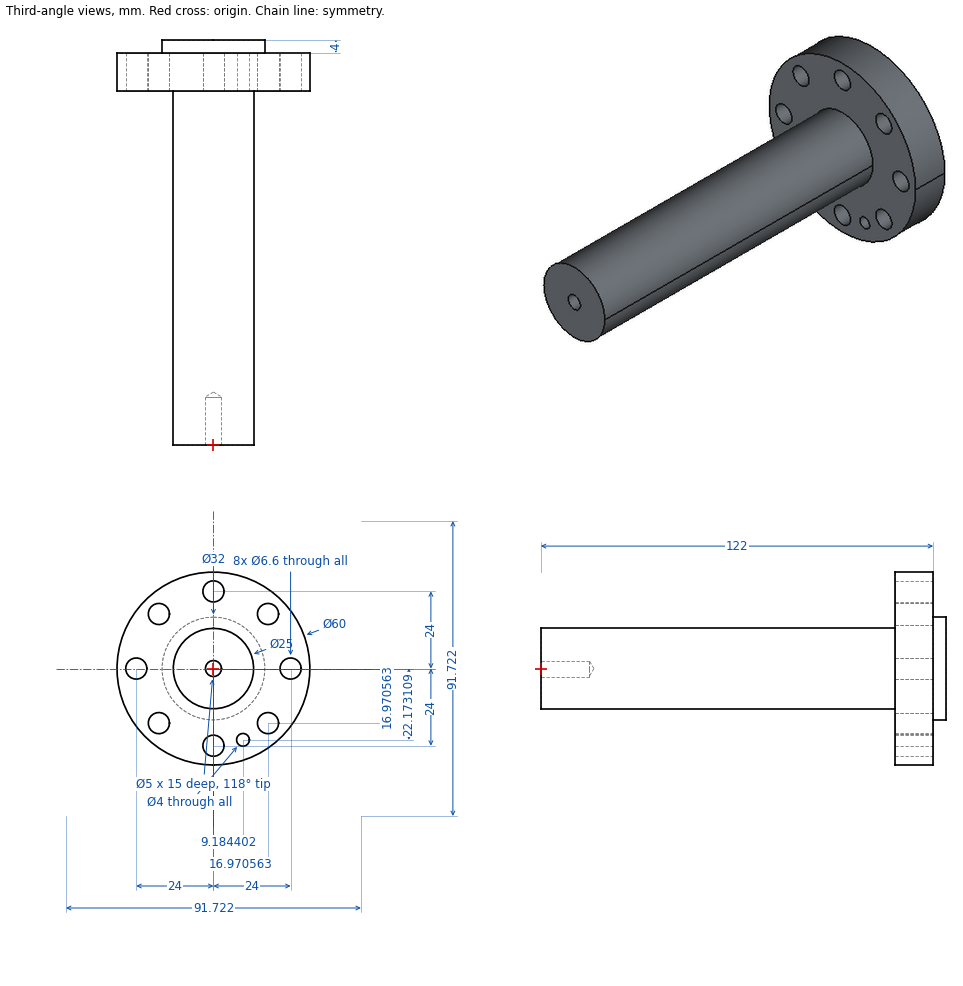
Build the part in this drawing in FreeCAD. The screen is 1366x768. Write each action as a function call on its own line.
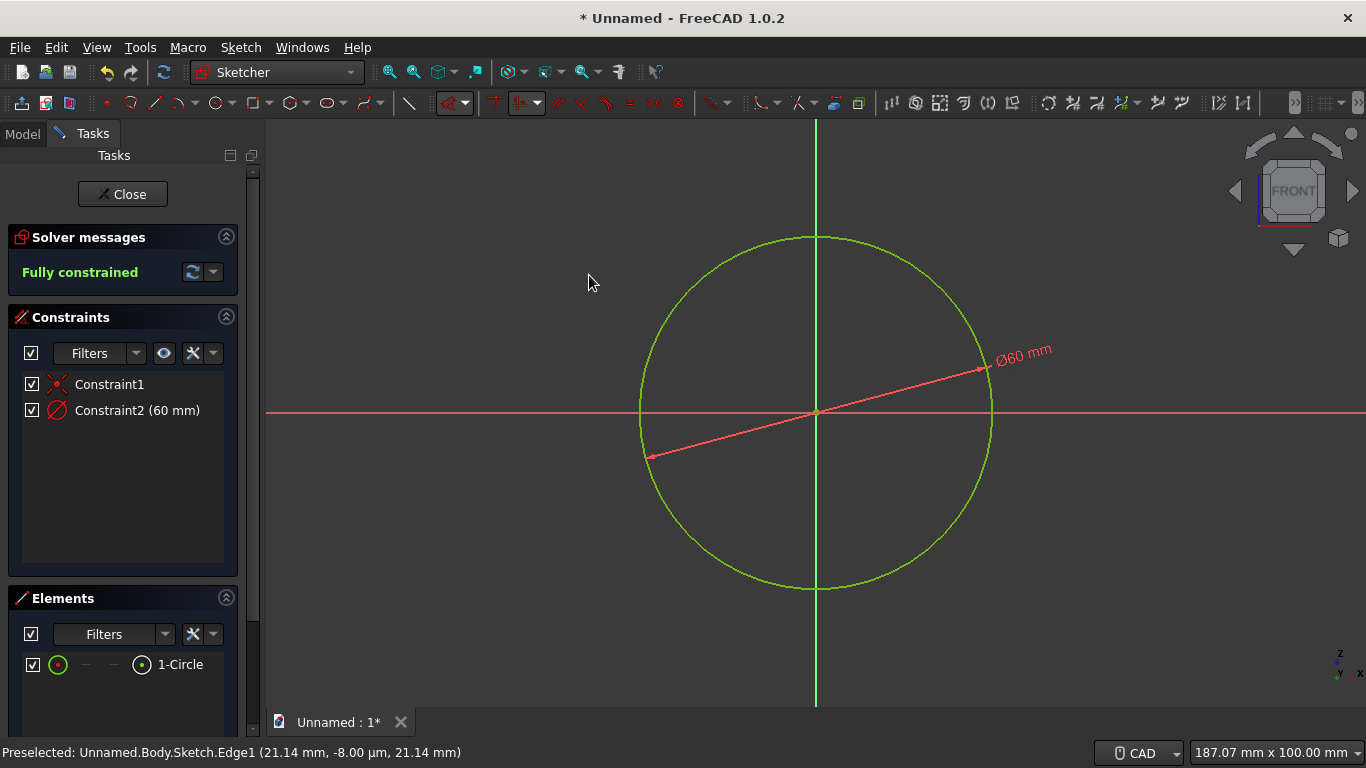
click(123, 194)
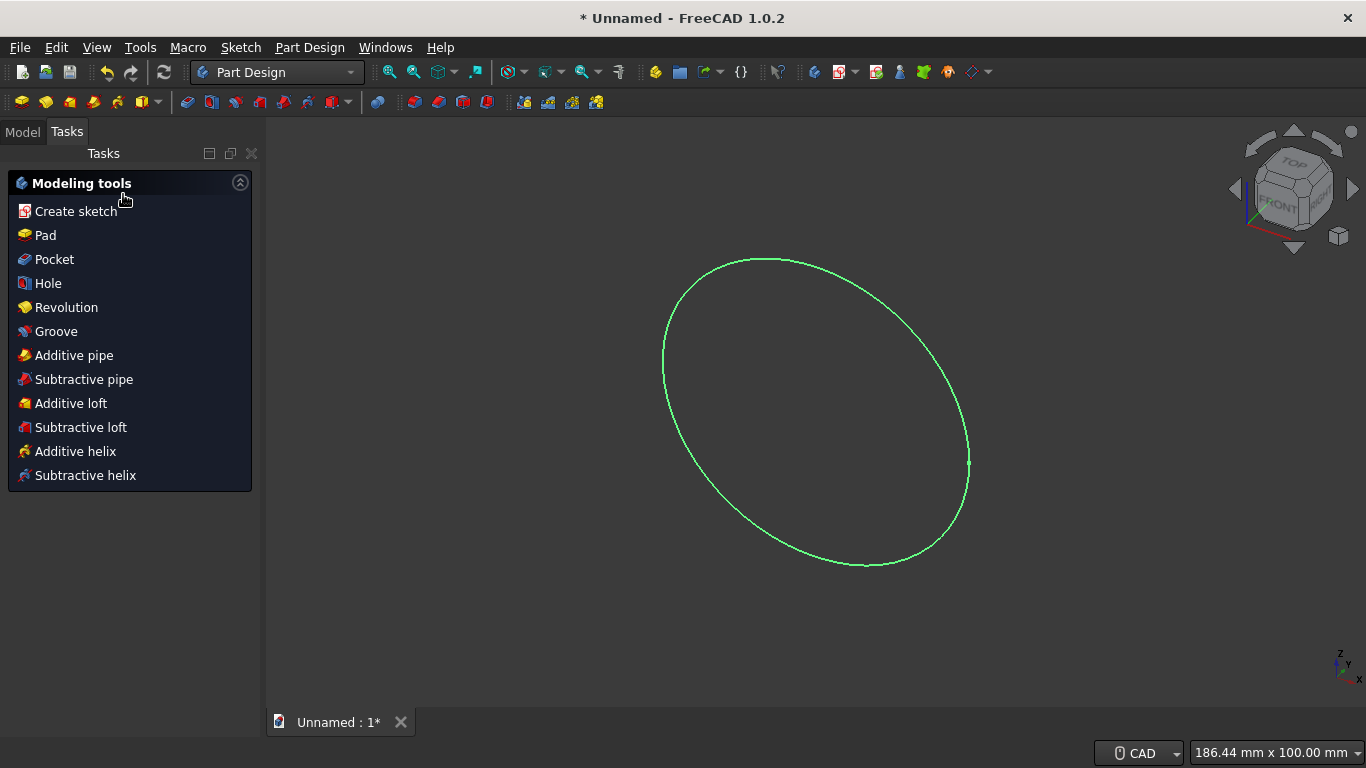
click(22, 102)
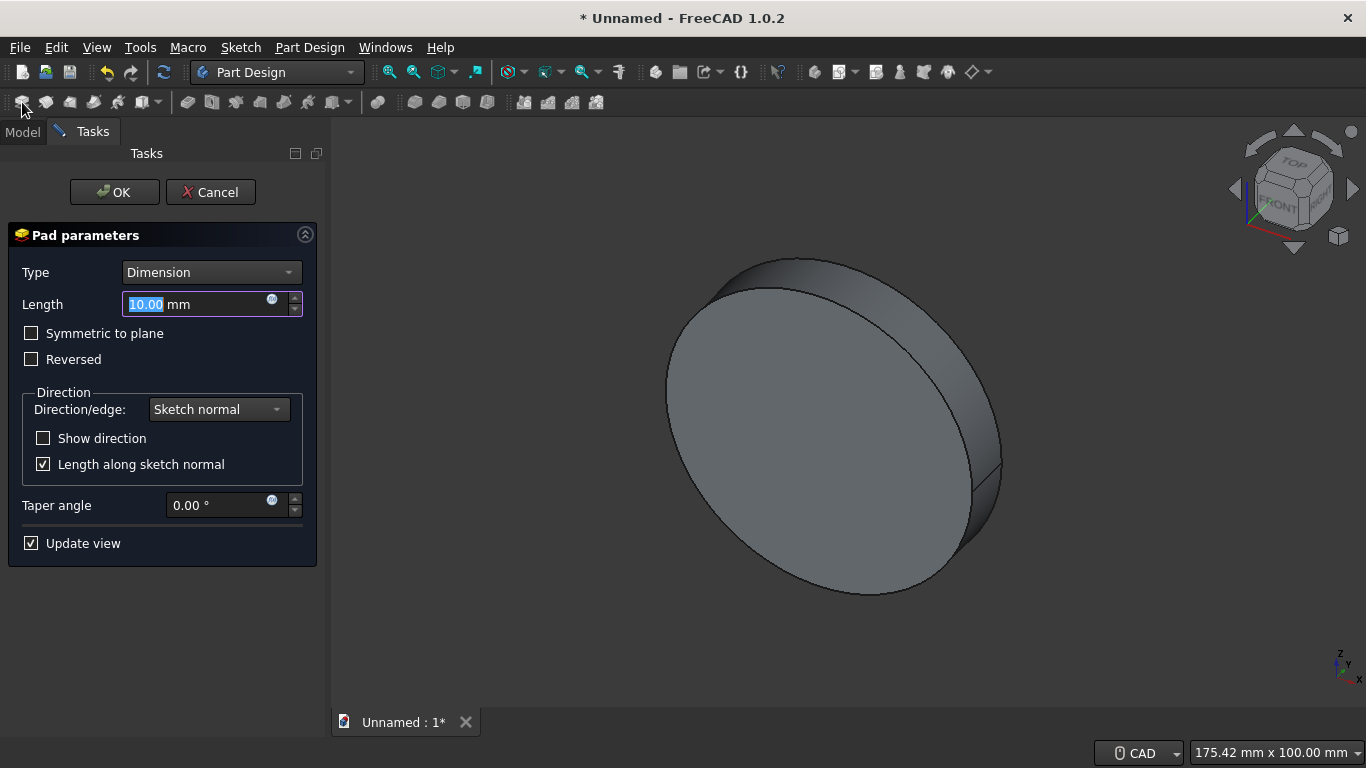
text(122)
key(Tab)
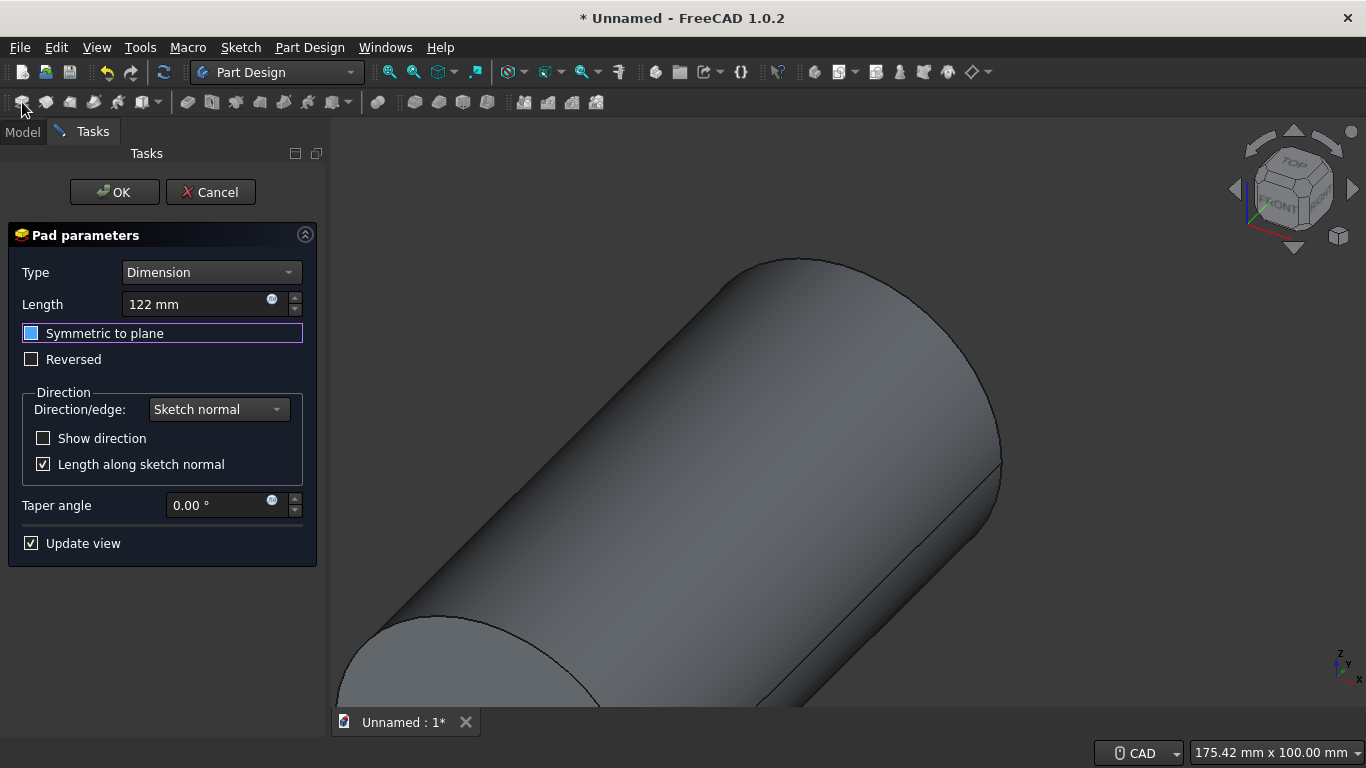
click(30, 359)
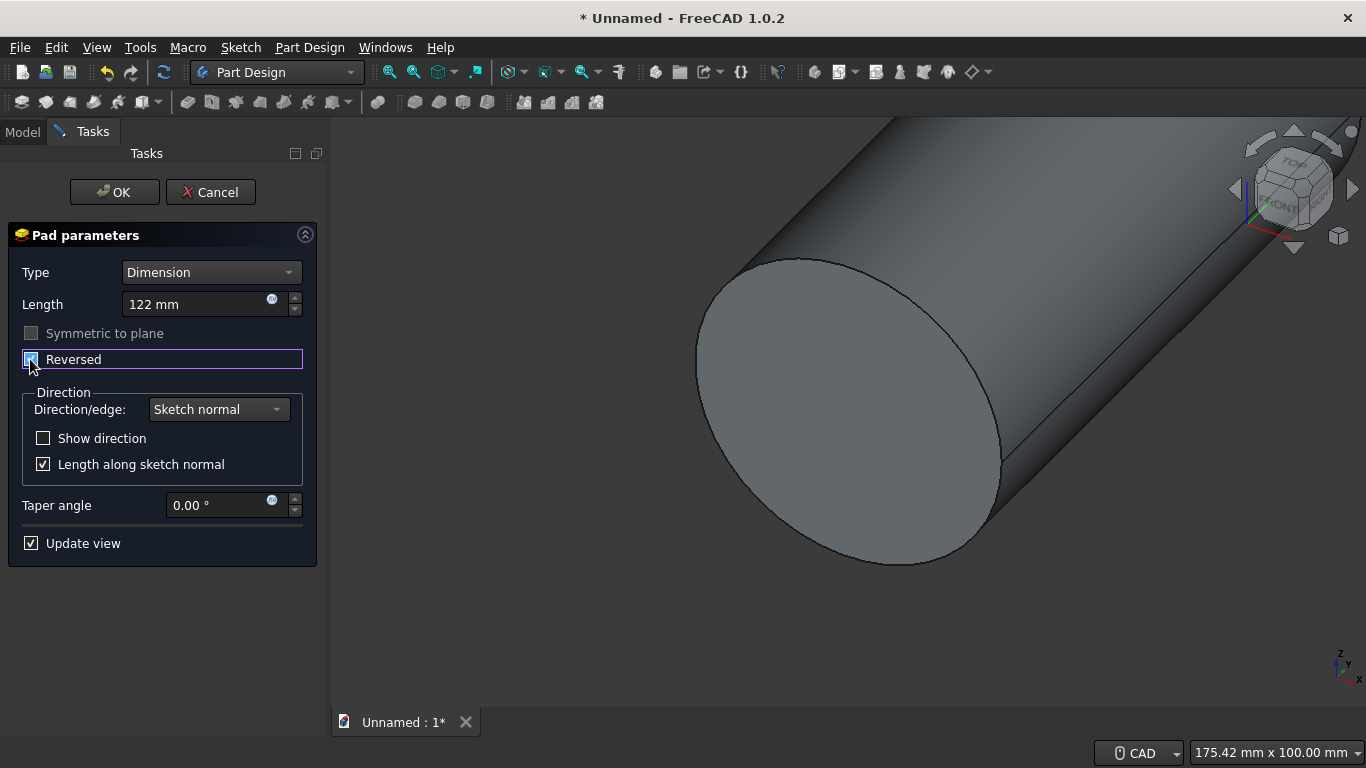
click(115, 192)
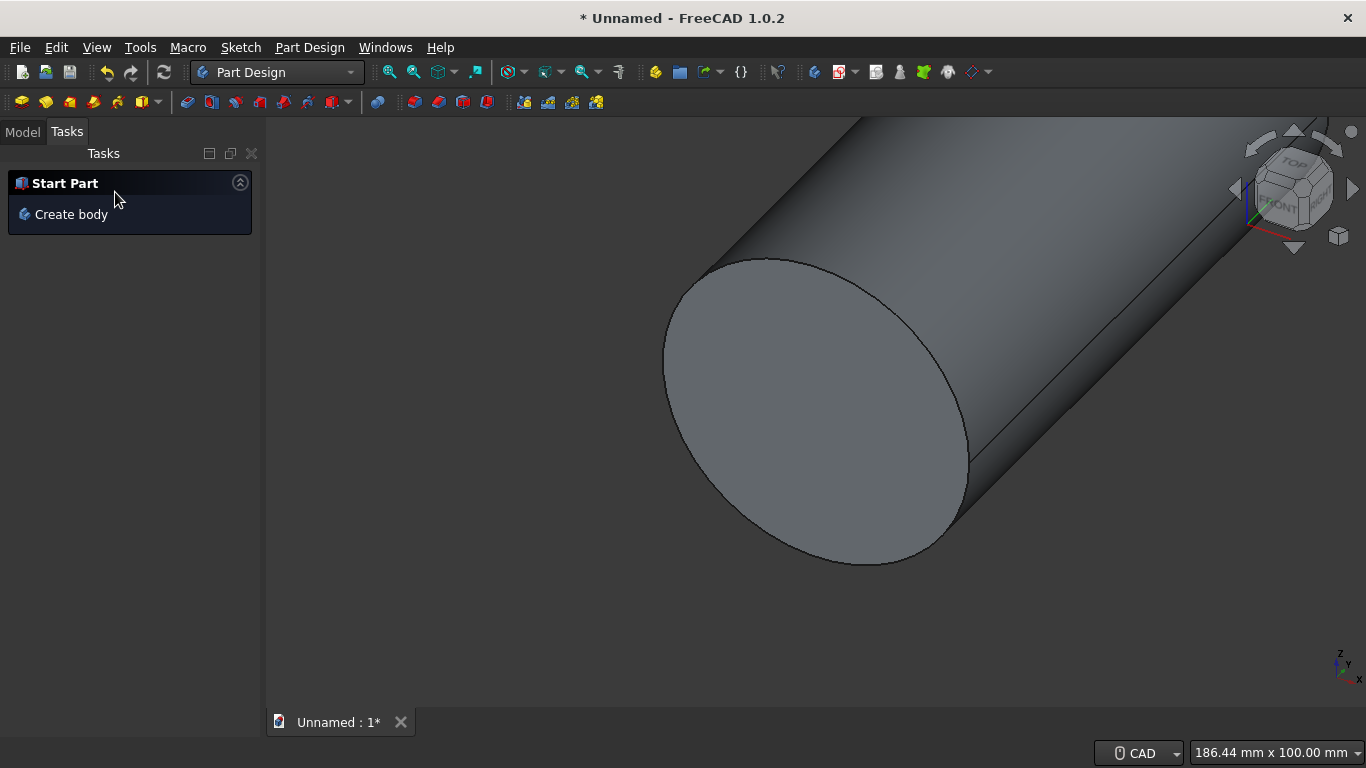
click(390, 72)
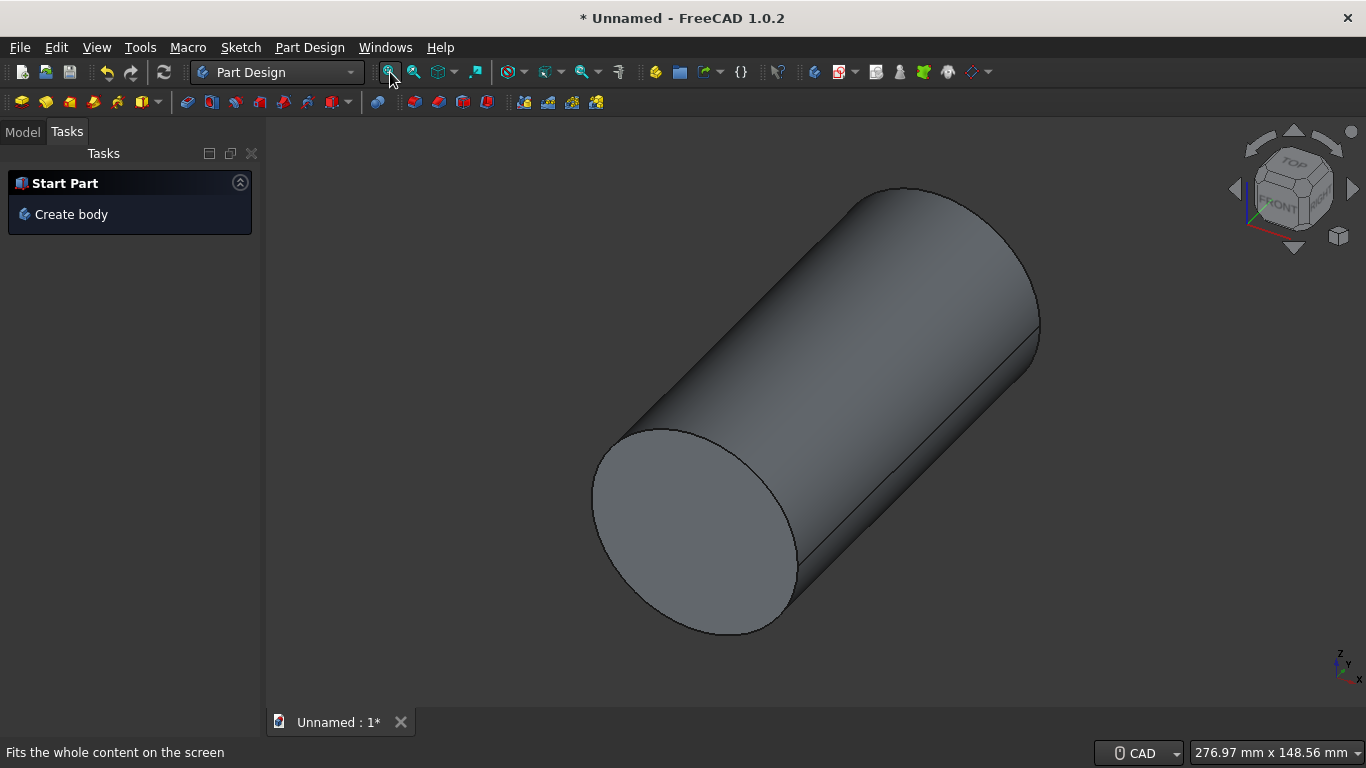
click(23, 131)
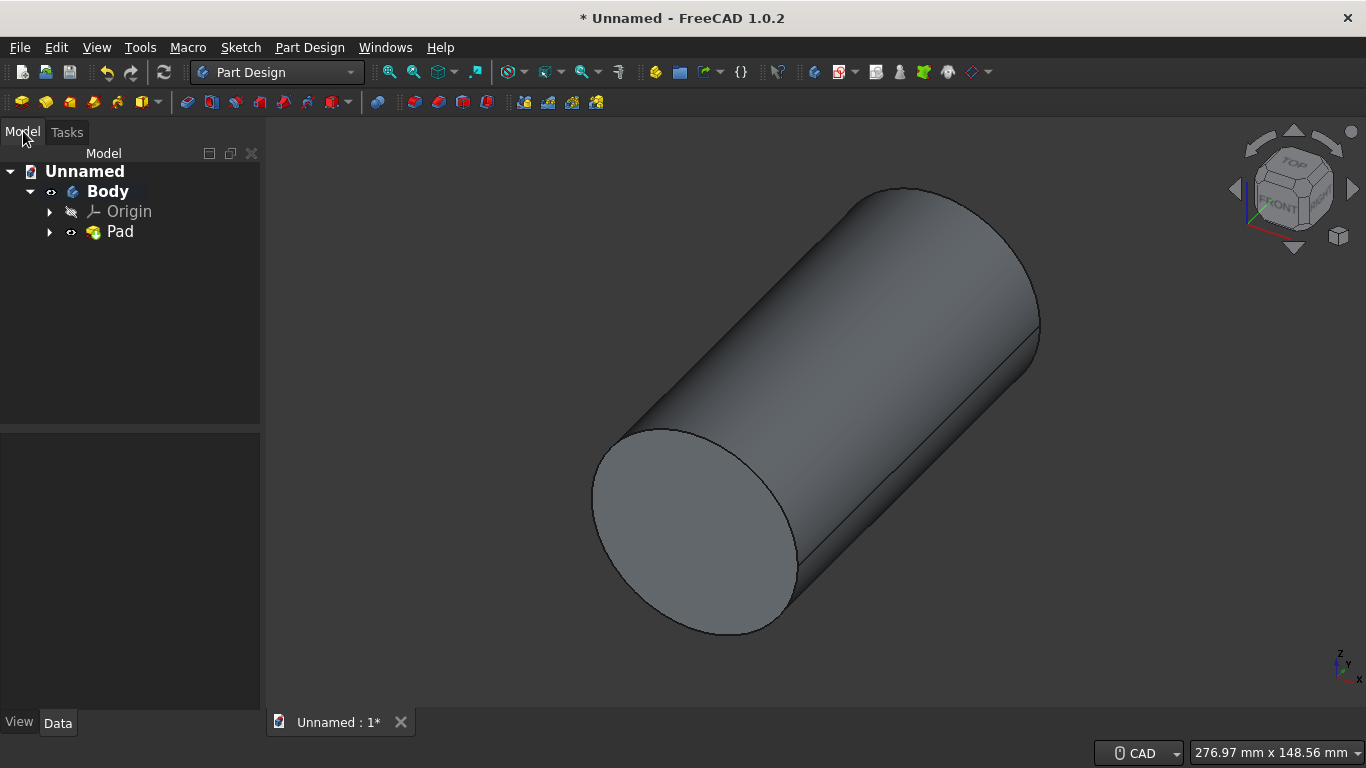
click(50, 212)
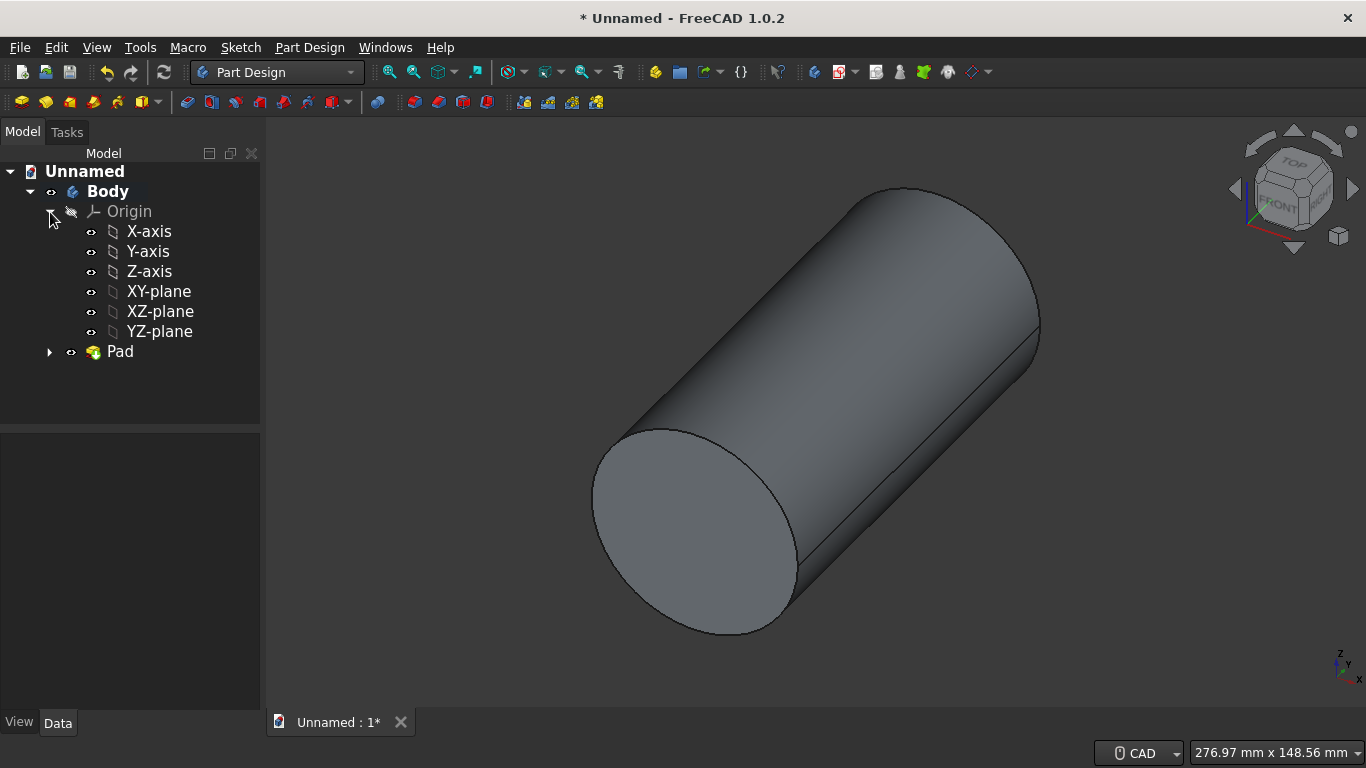
click(136, 312)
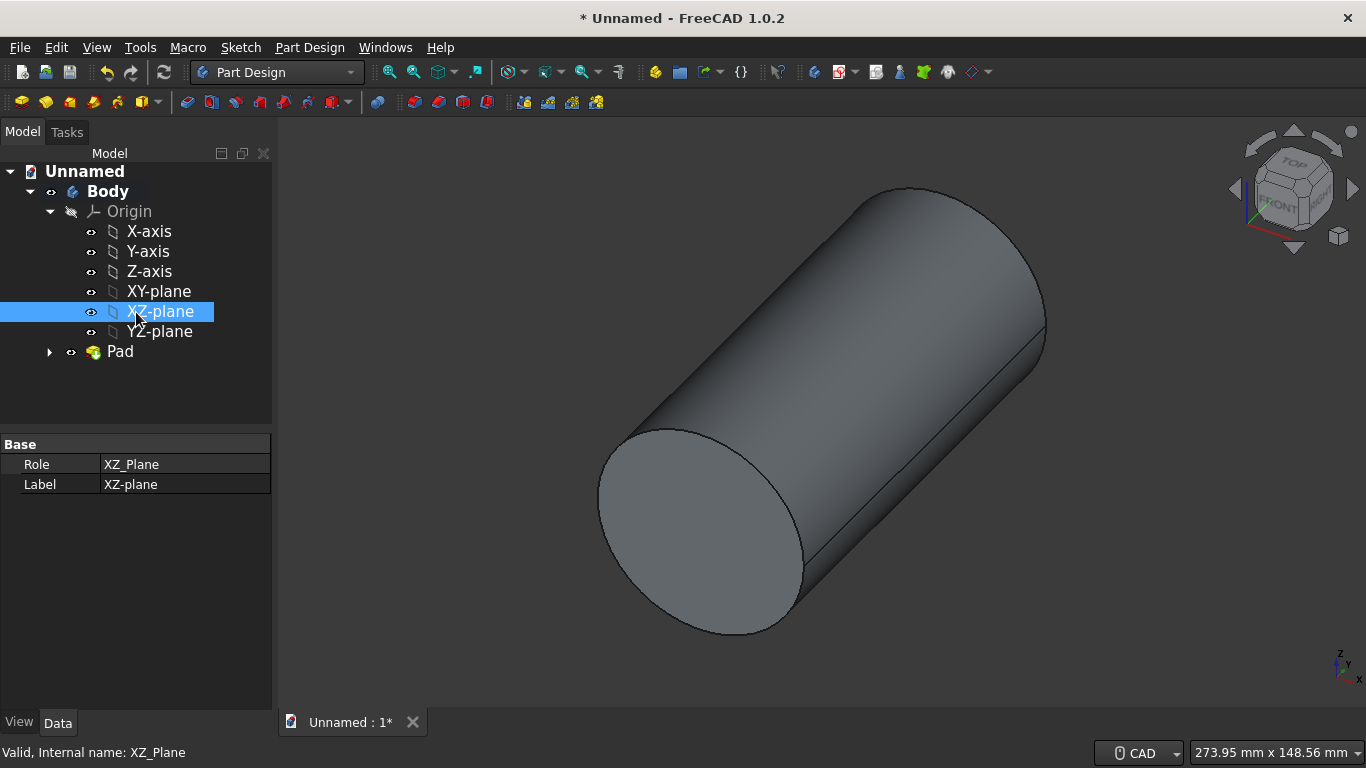
click(972, 72)